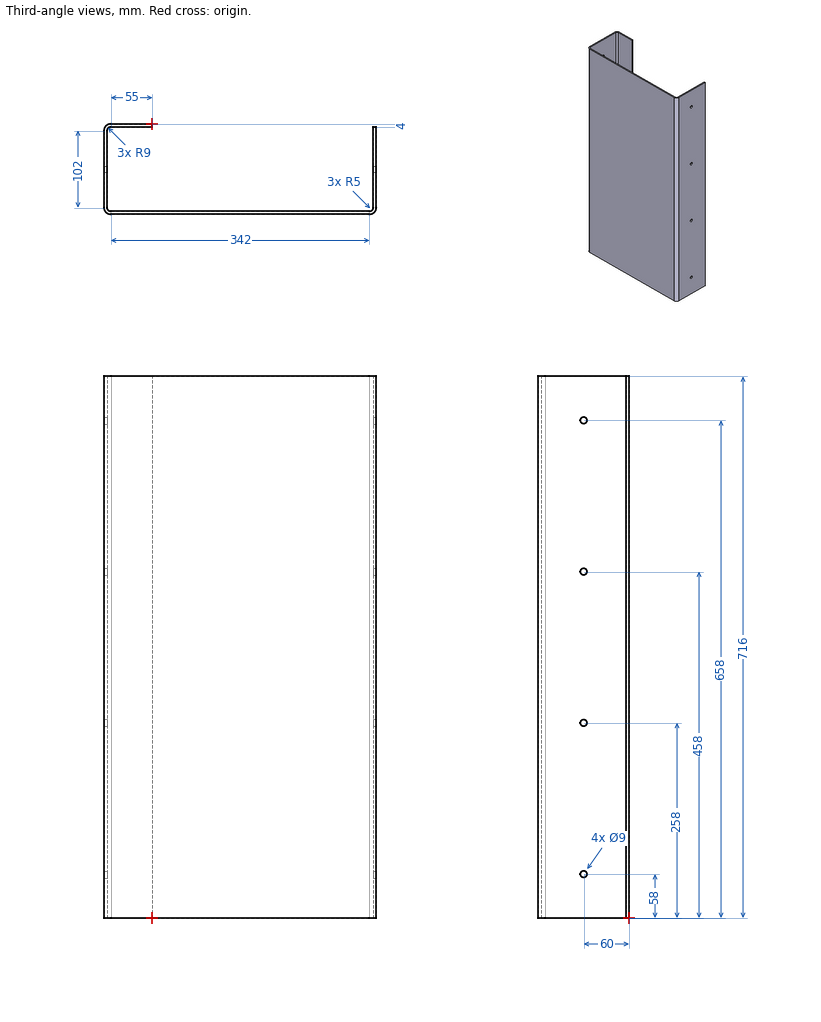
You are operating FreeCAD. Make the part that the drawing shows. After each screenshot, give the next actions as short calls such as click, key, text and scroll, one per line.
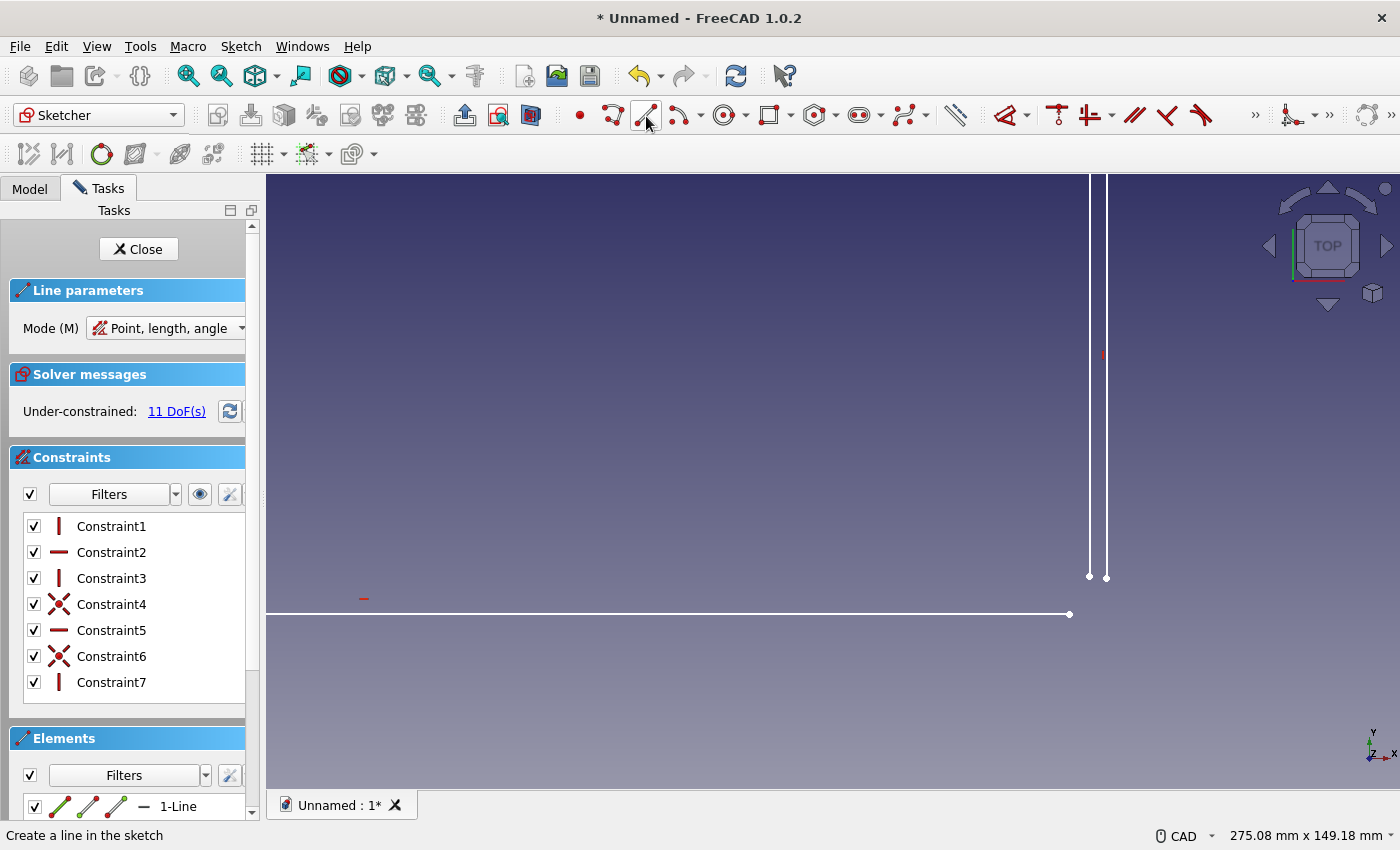
click(1069, 597)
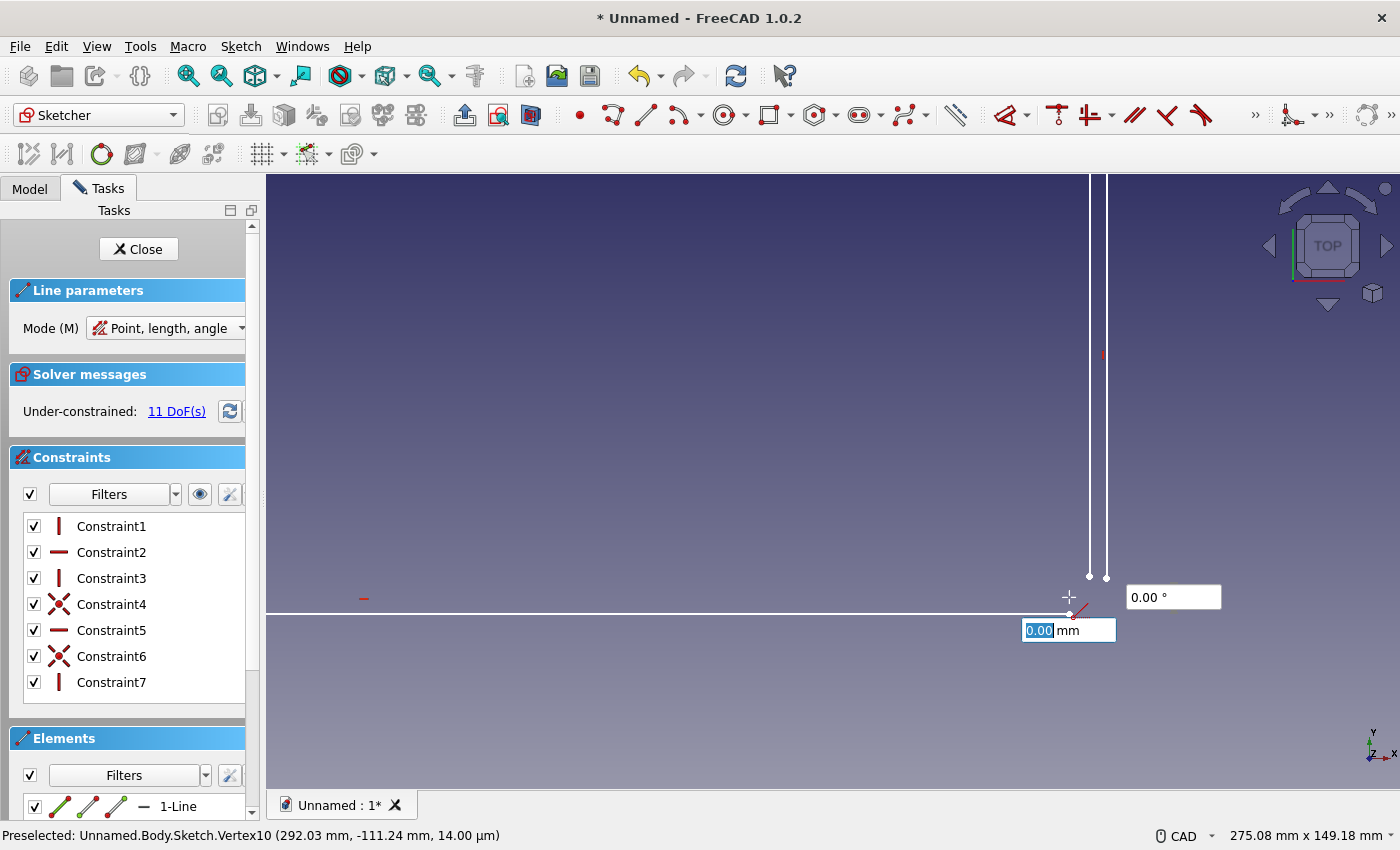
scroll(1091, 576, down, 4)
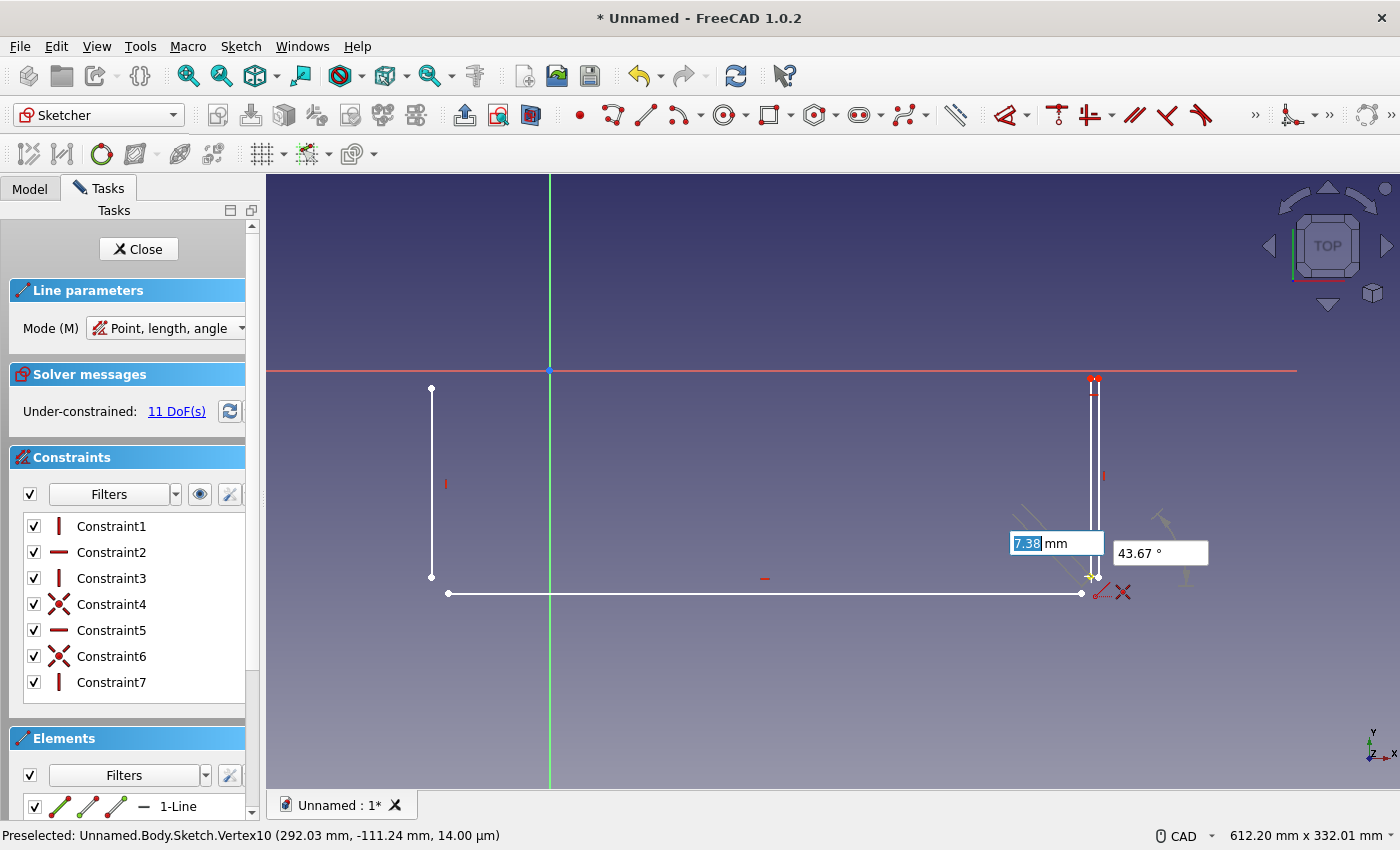
scroll(448, 586, up, 4)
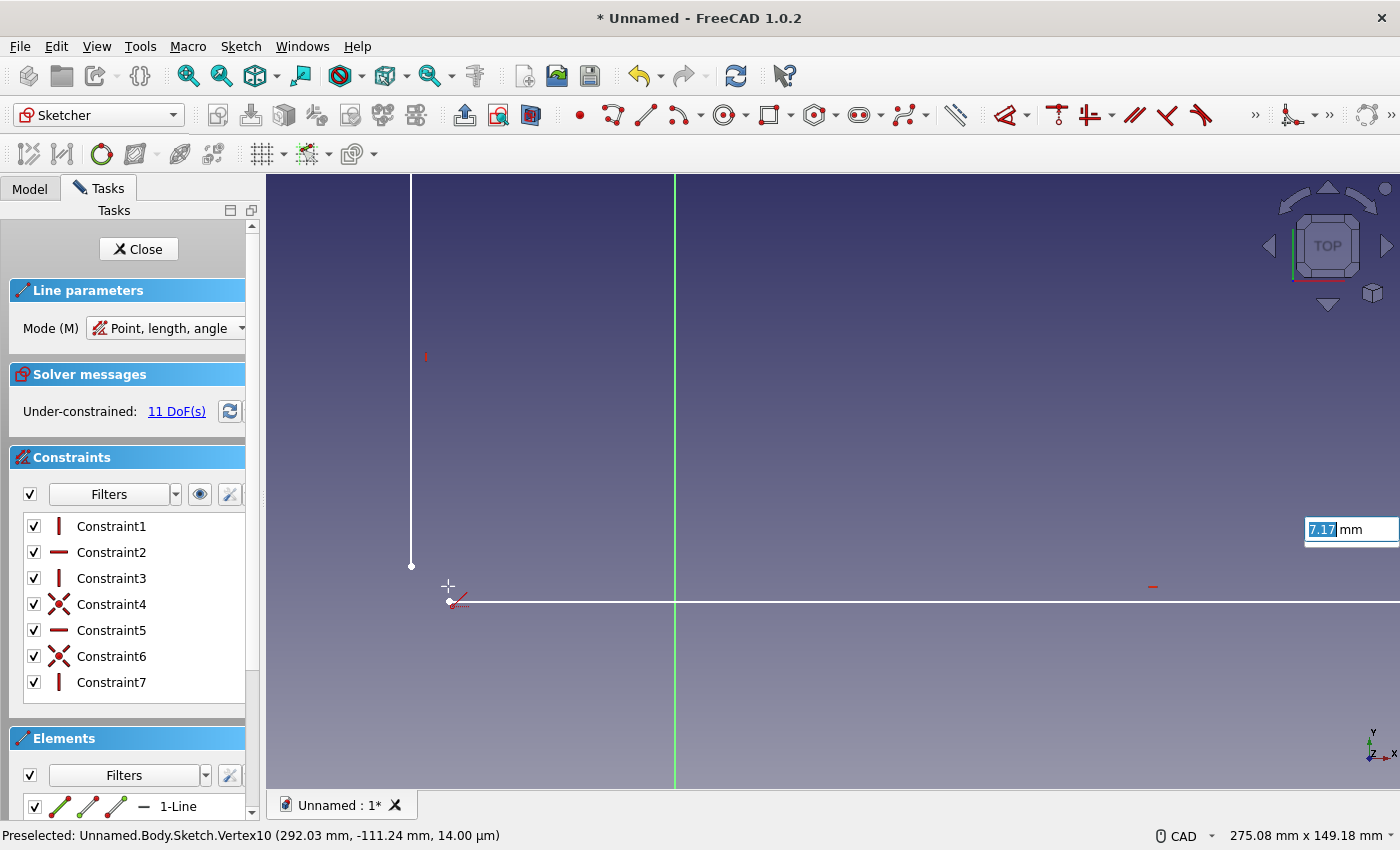
click(448, 585)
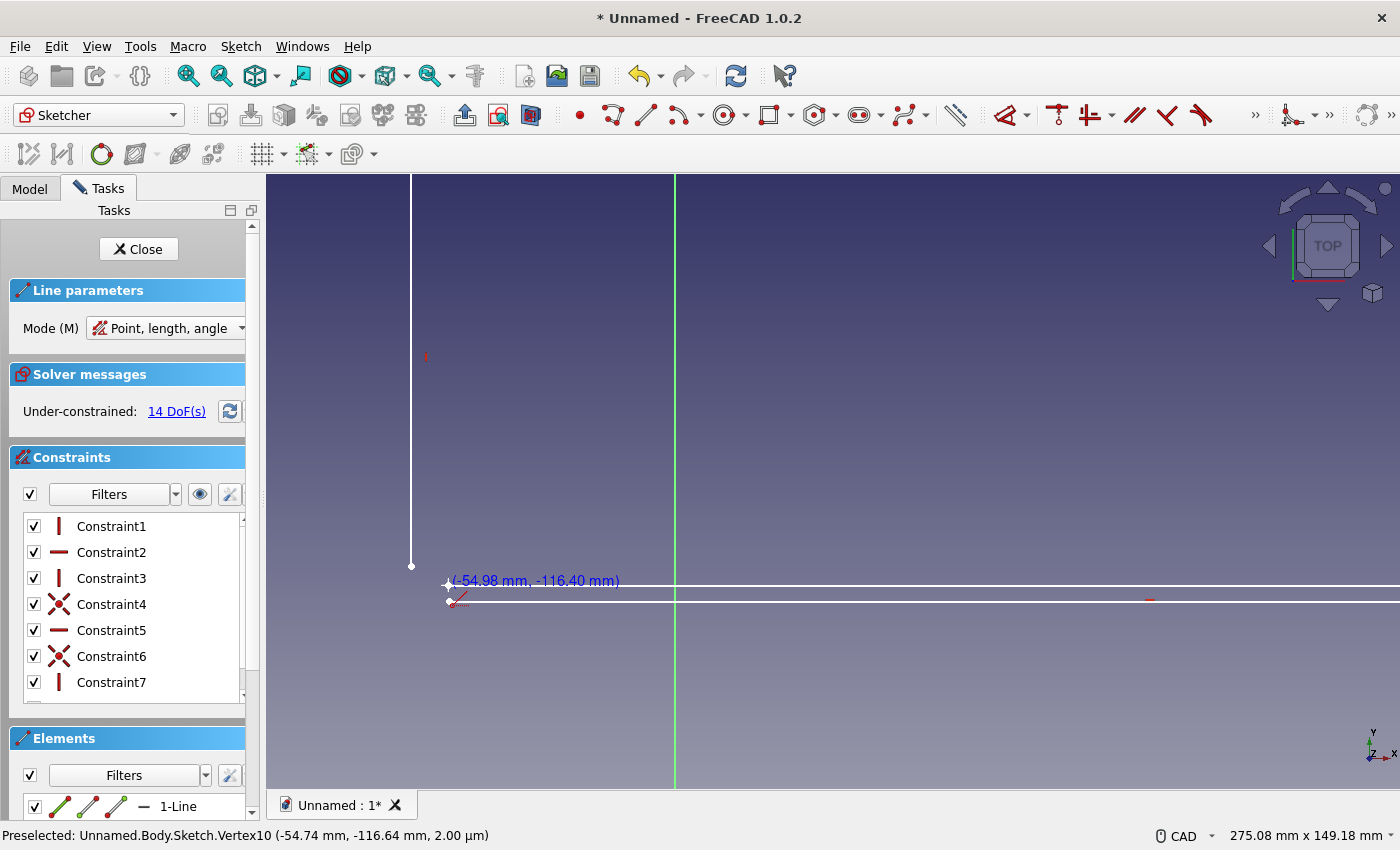
click(427, 564)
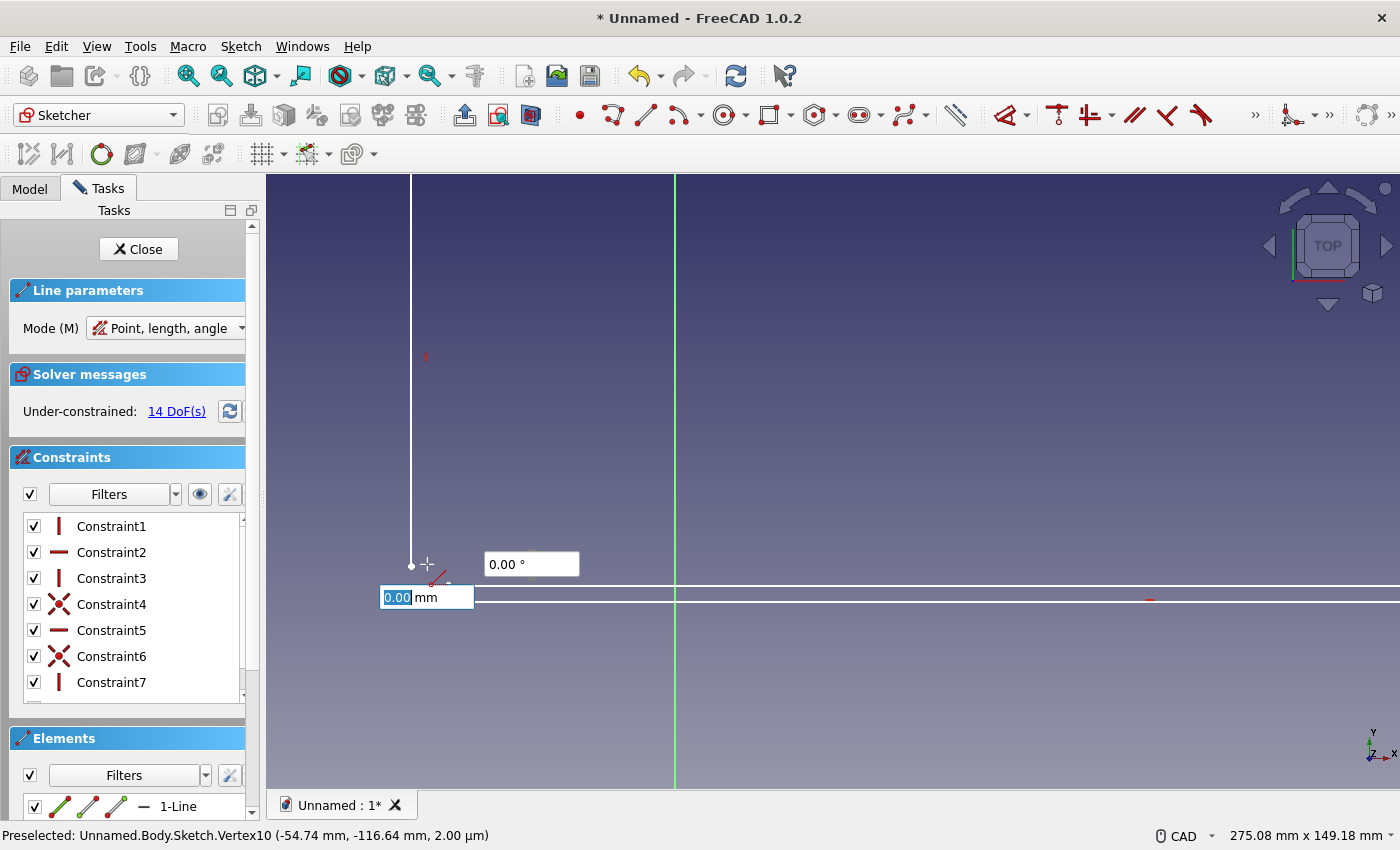
scroll(448, 586, down, 4)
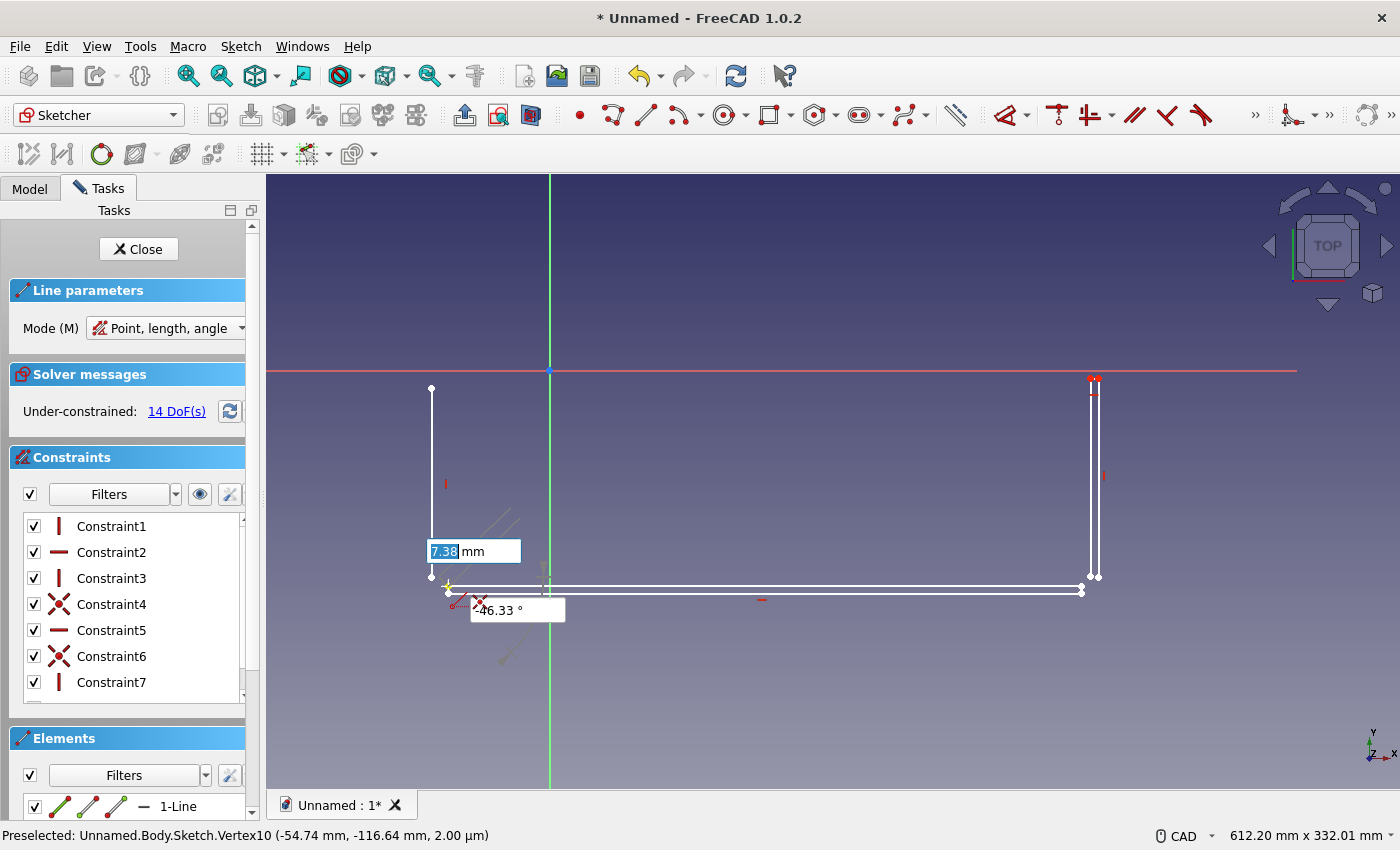
scroll(439, 387, up, 4)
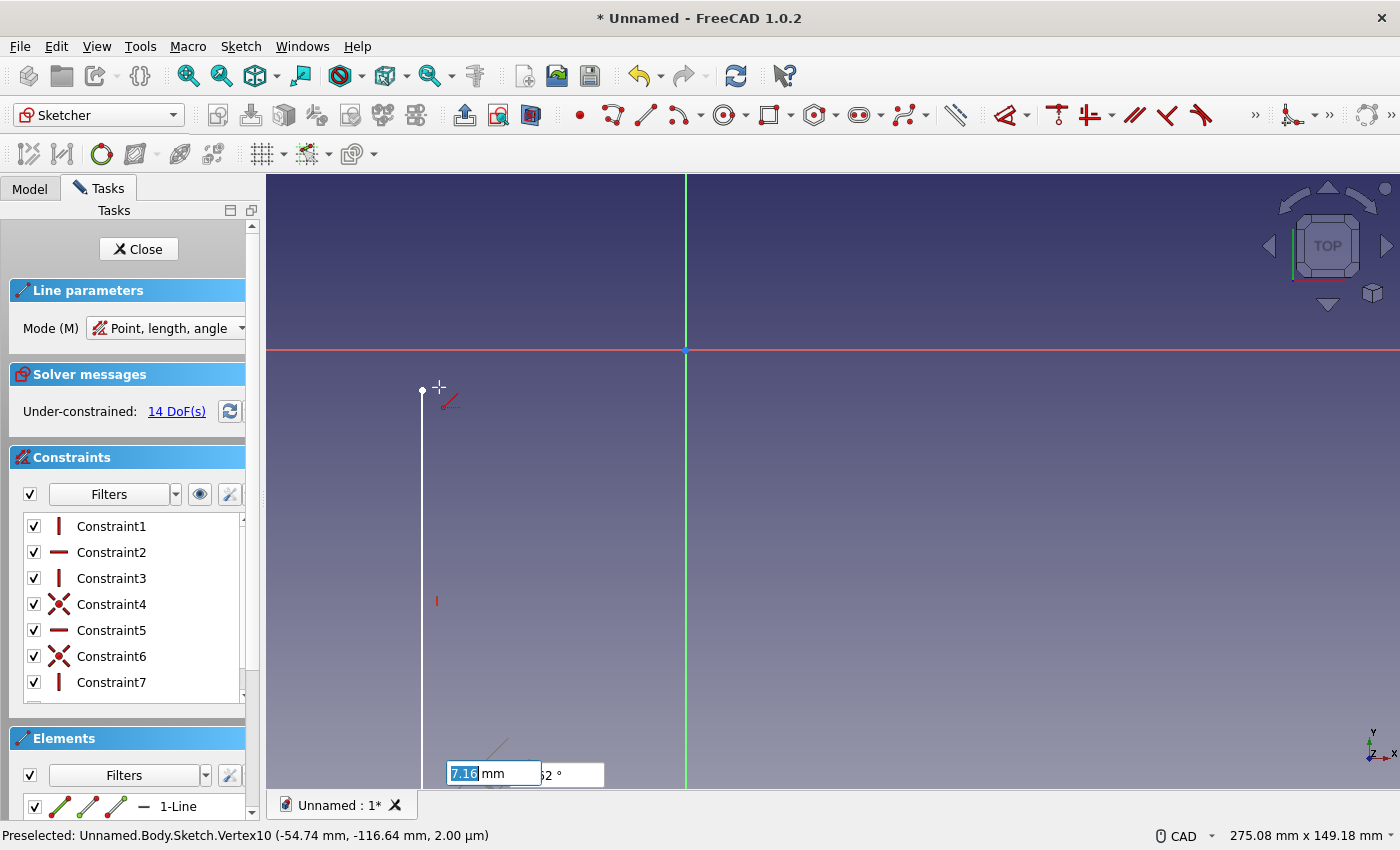
click(438, 388)